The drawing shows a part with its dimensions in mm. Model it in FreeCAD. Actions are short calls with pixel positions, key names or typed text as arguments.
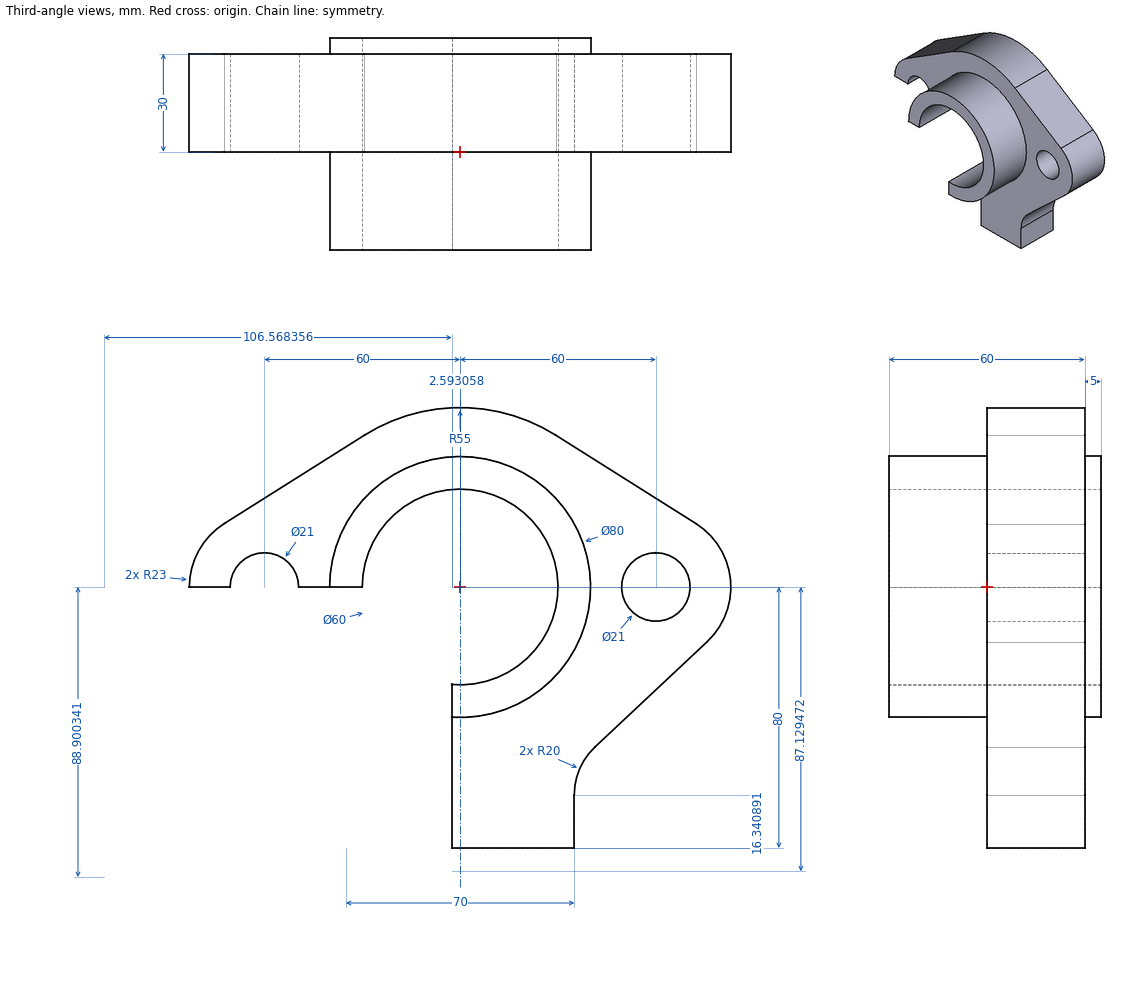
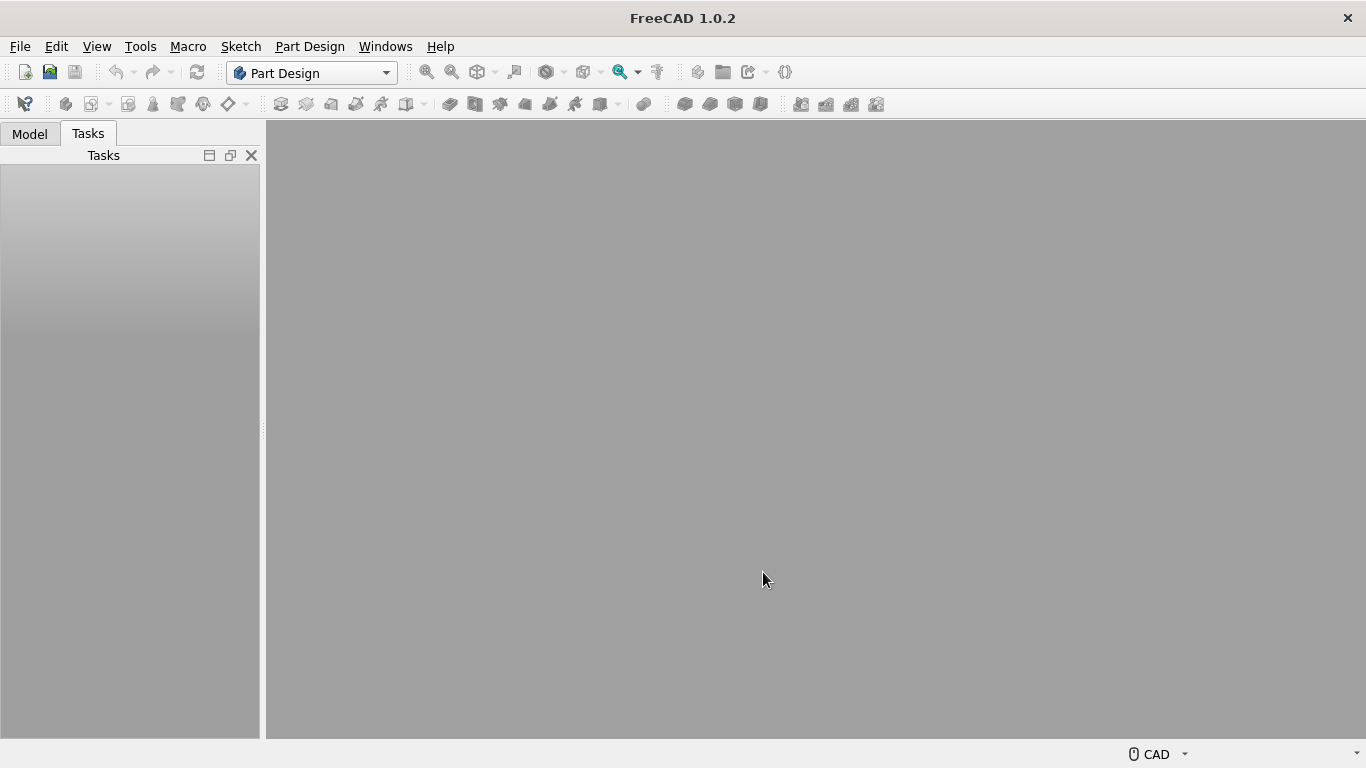
click(25, 72)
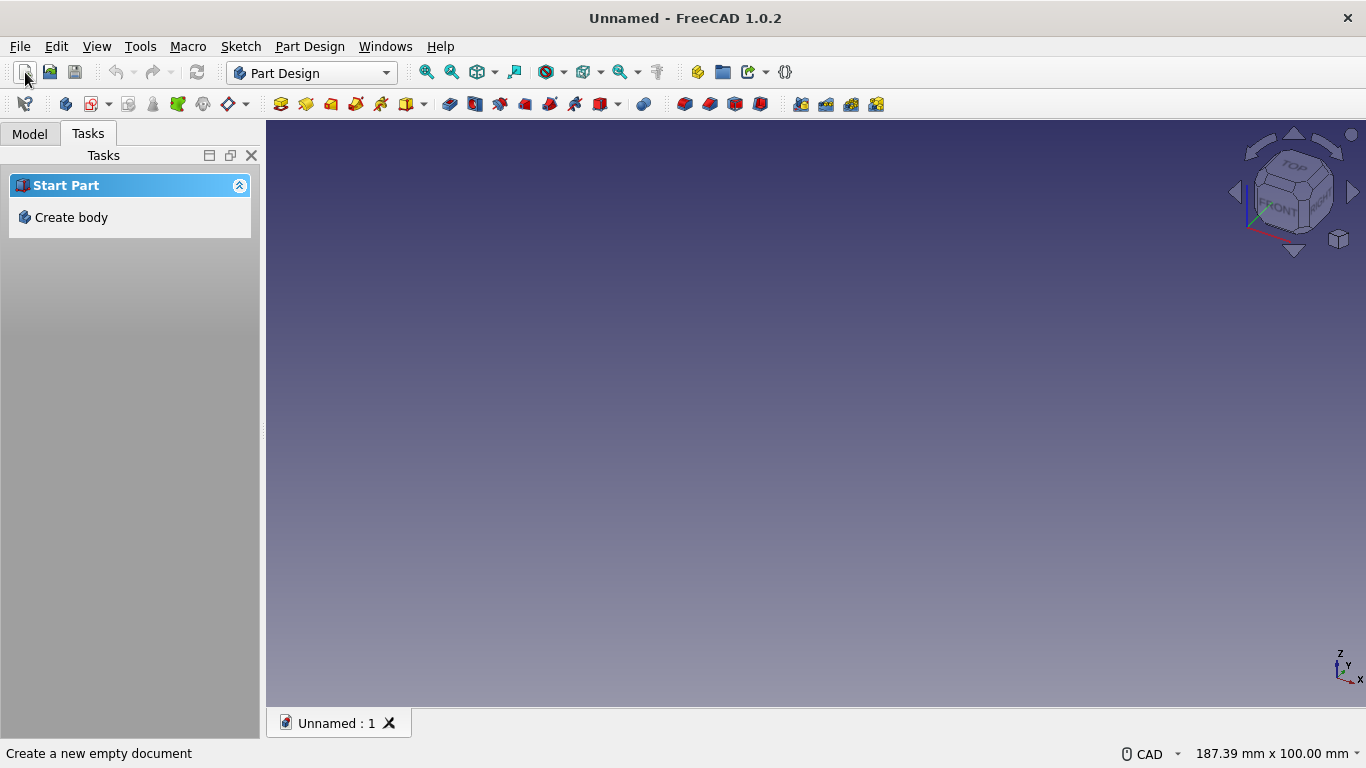
click(90, 104)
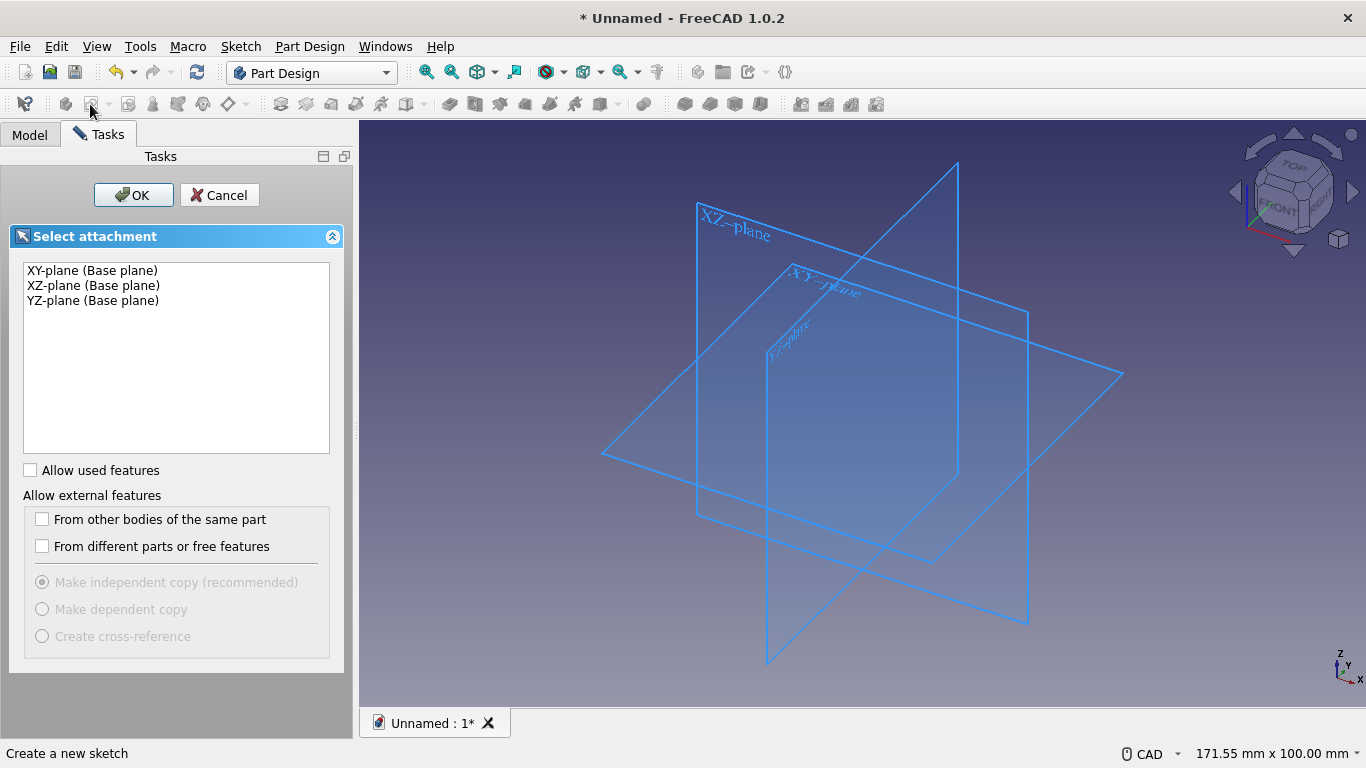
click(84, 286)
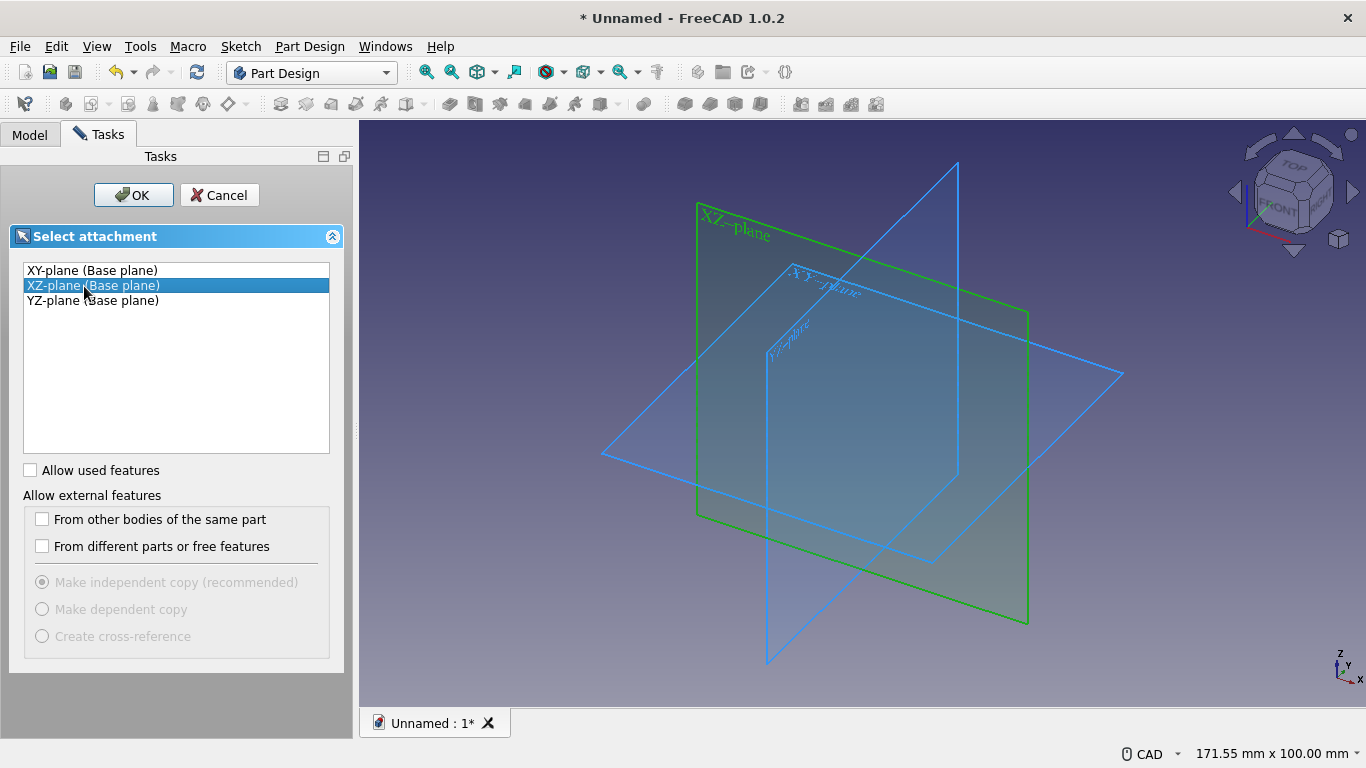
click(134, 195)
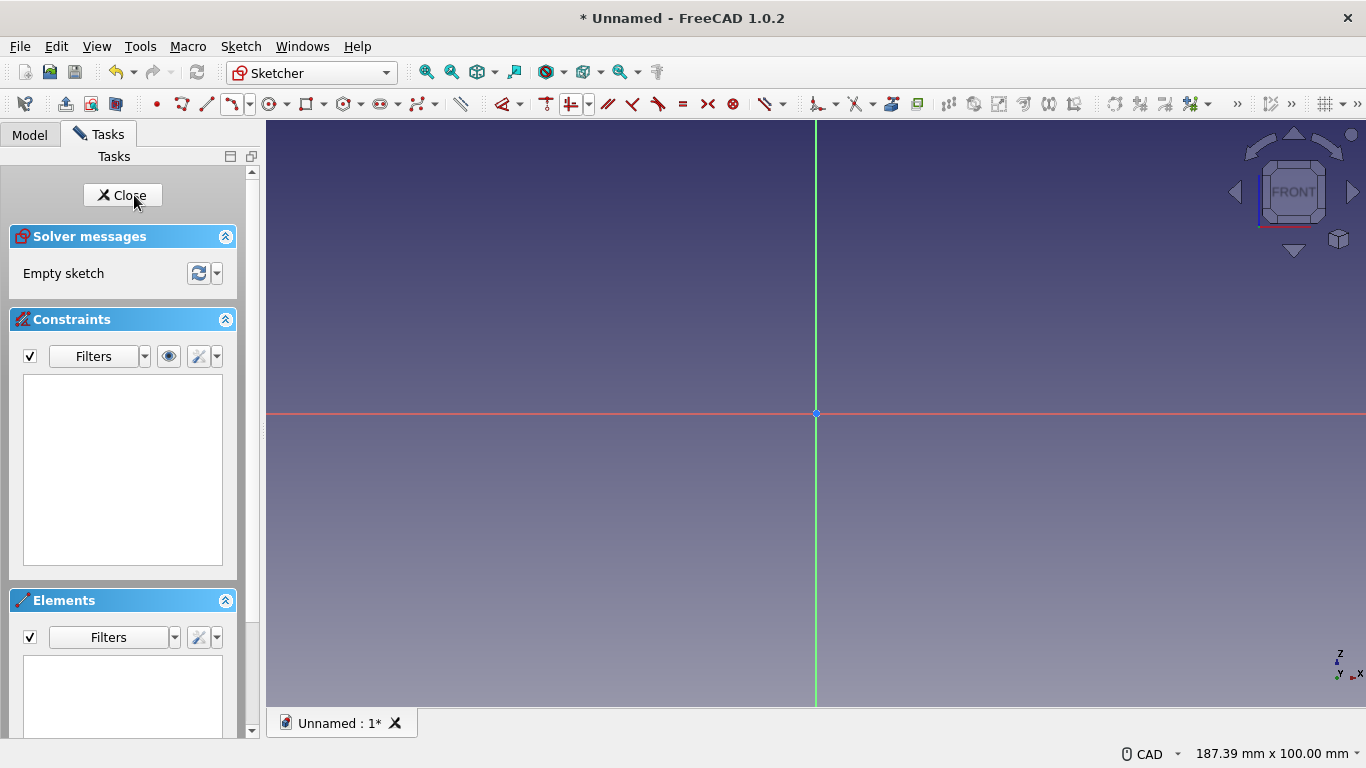
click(268, 104)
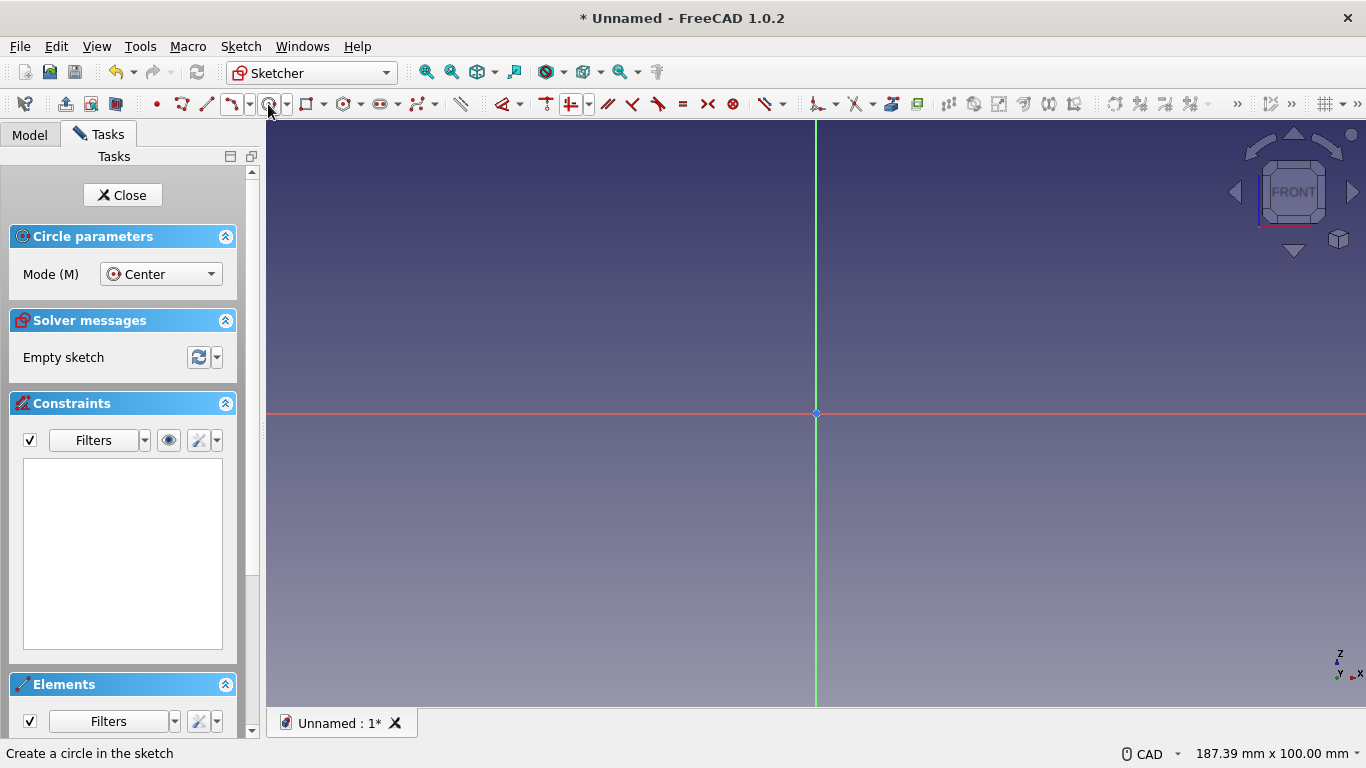
click(816, 414)
move(982, 247)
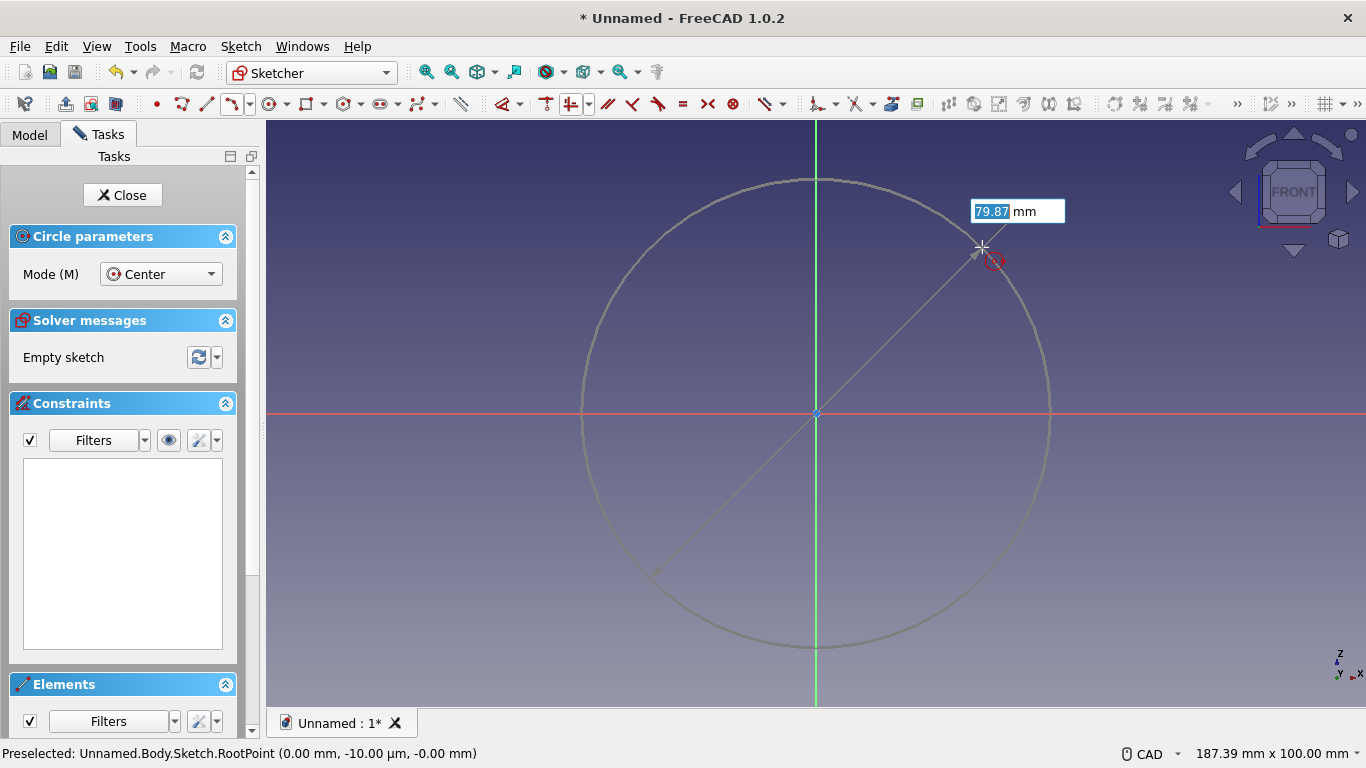
text(80)
key(Return)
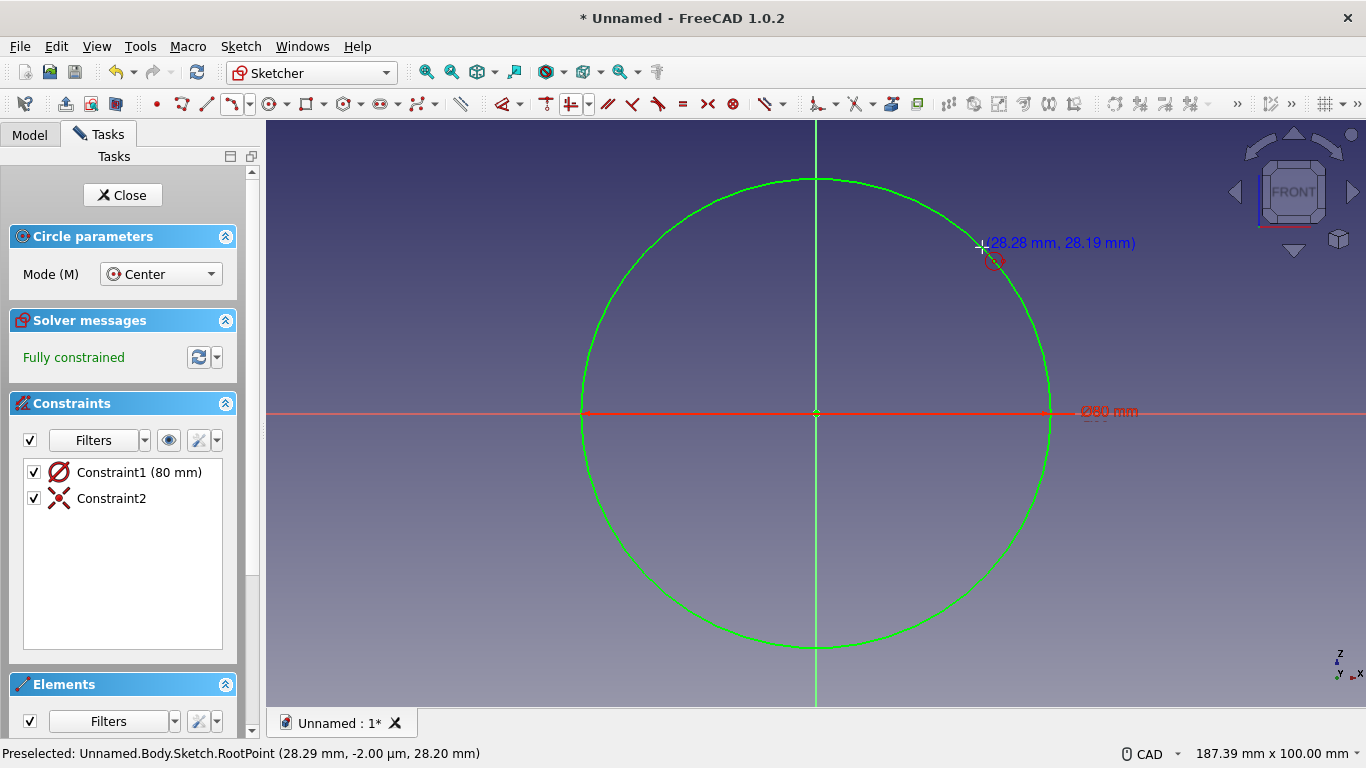
click(816, 414)
move(941, 289)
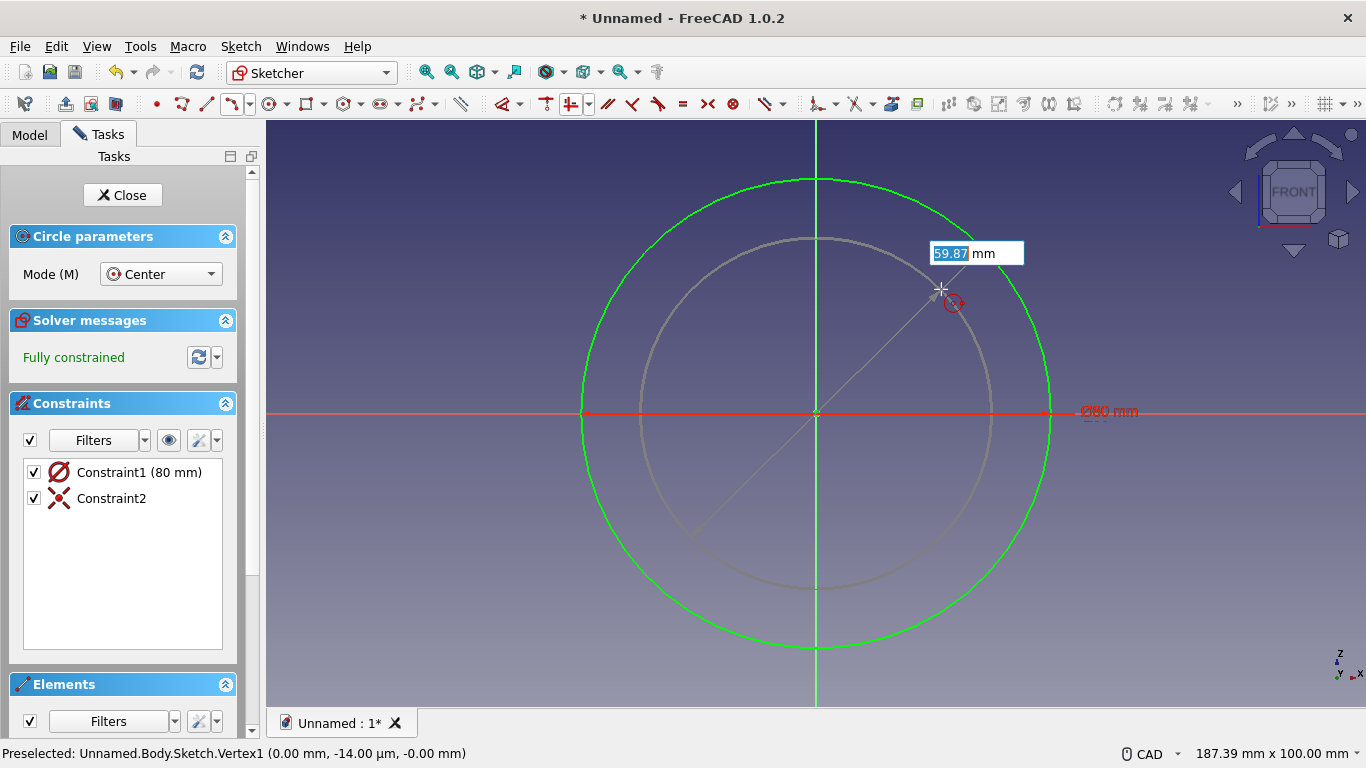
text(60)
key(Return)
key(Escape)